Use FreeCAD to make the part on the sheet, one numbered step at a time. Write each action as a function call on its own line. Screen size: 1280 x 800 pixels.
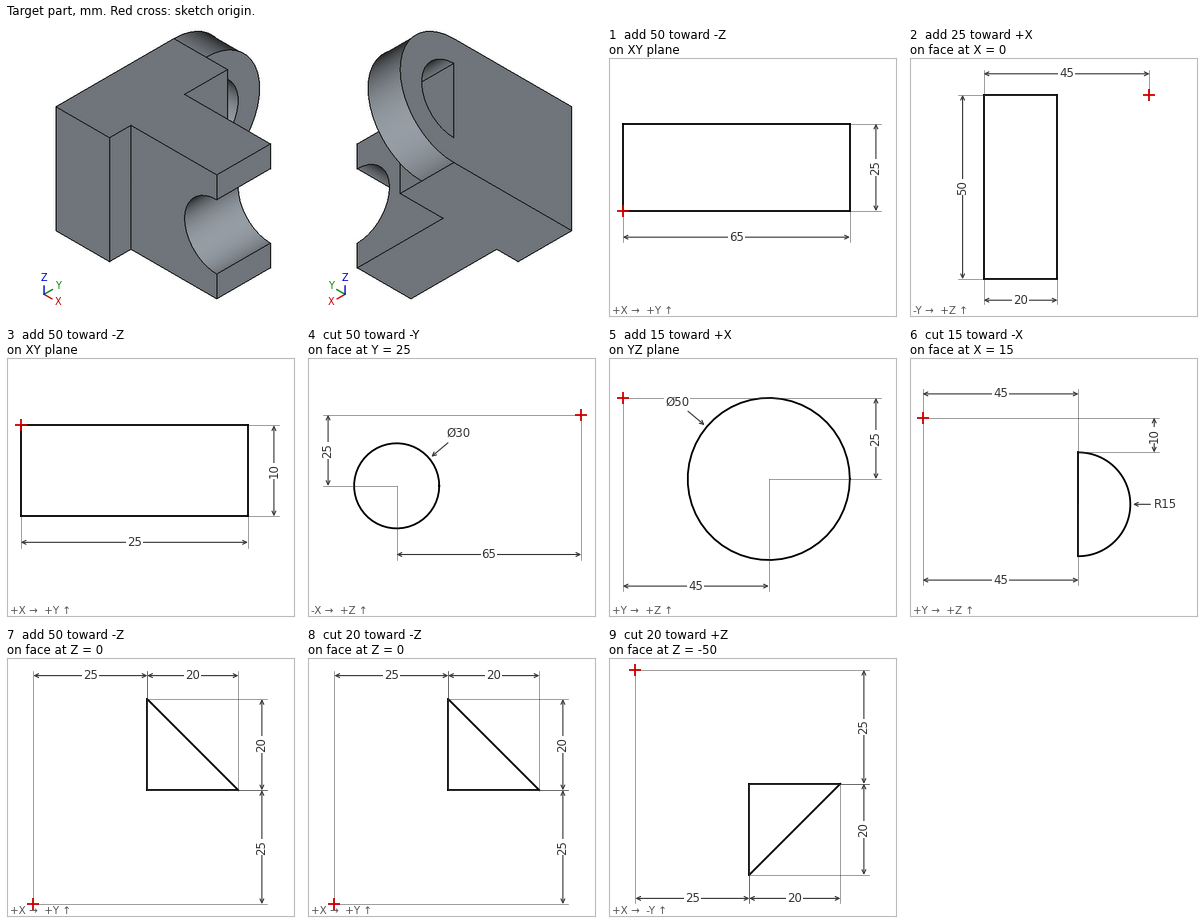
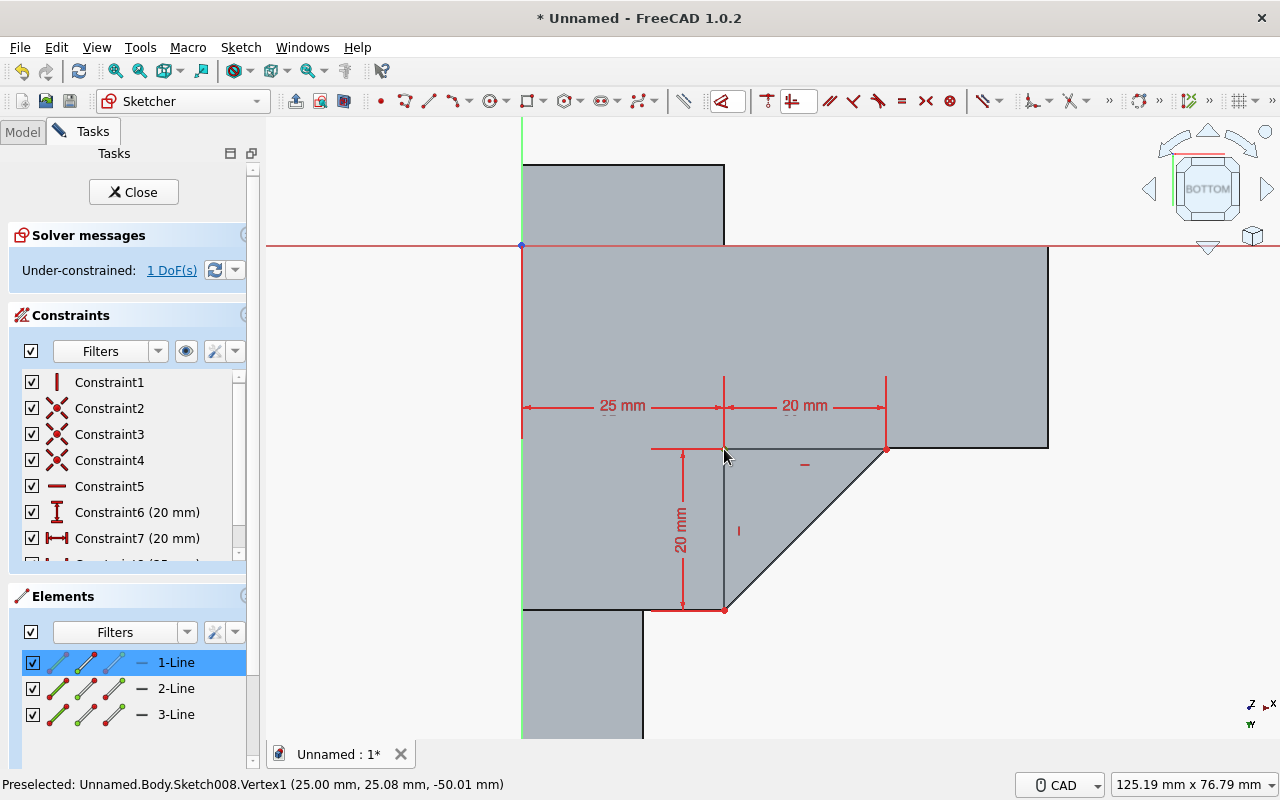
key(i)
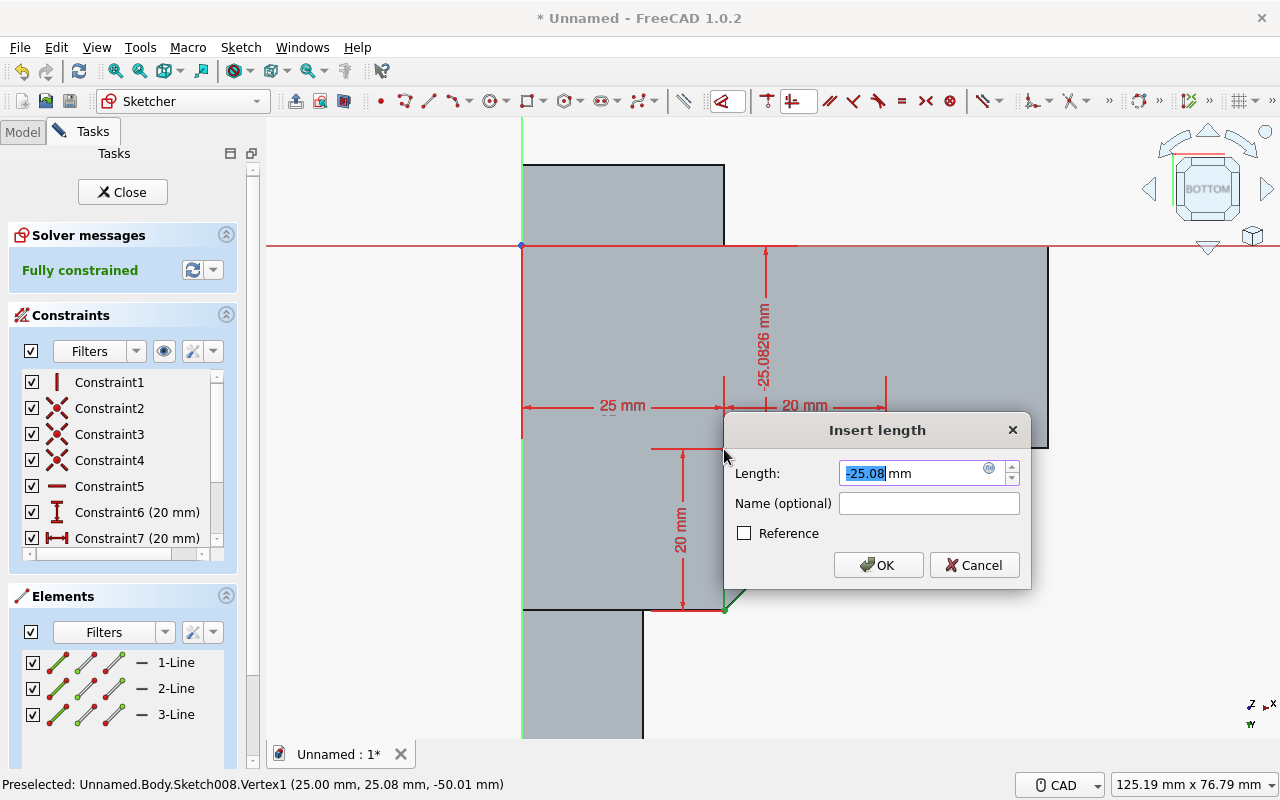
text(-25)
key(Return)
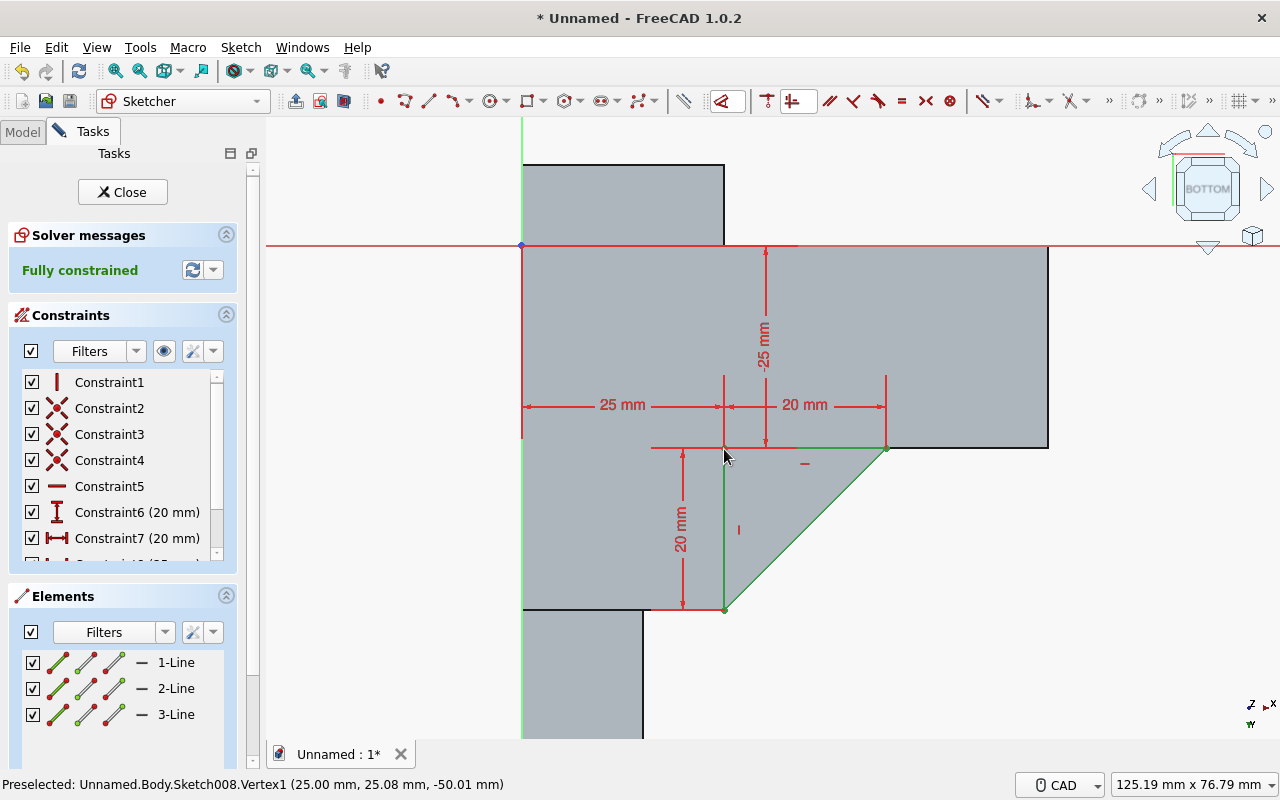
click(123, 192)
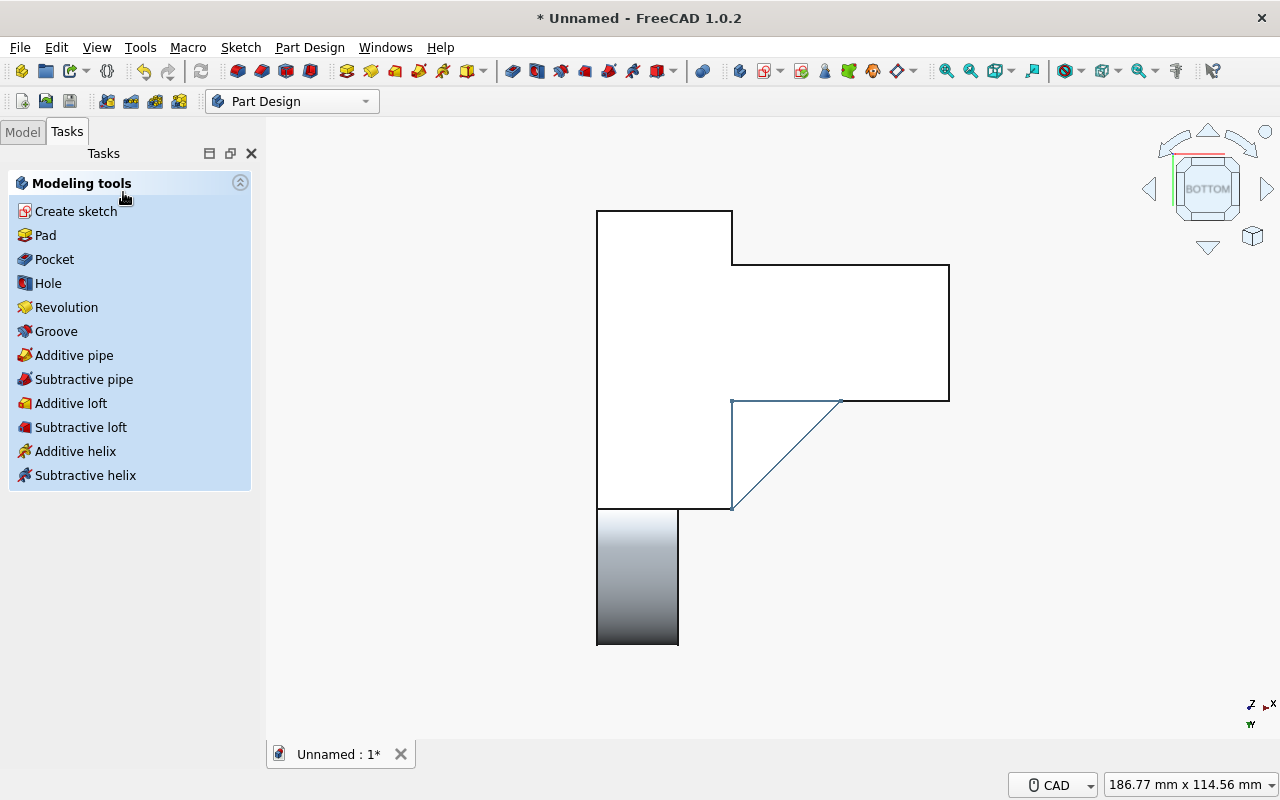
click(514, 72)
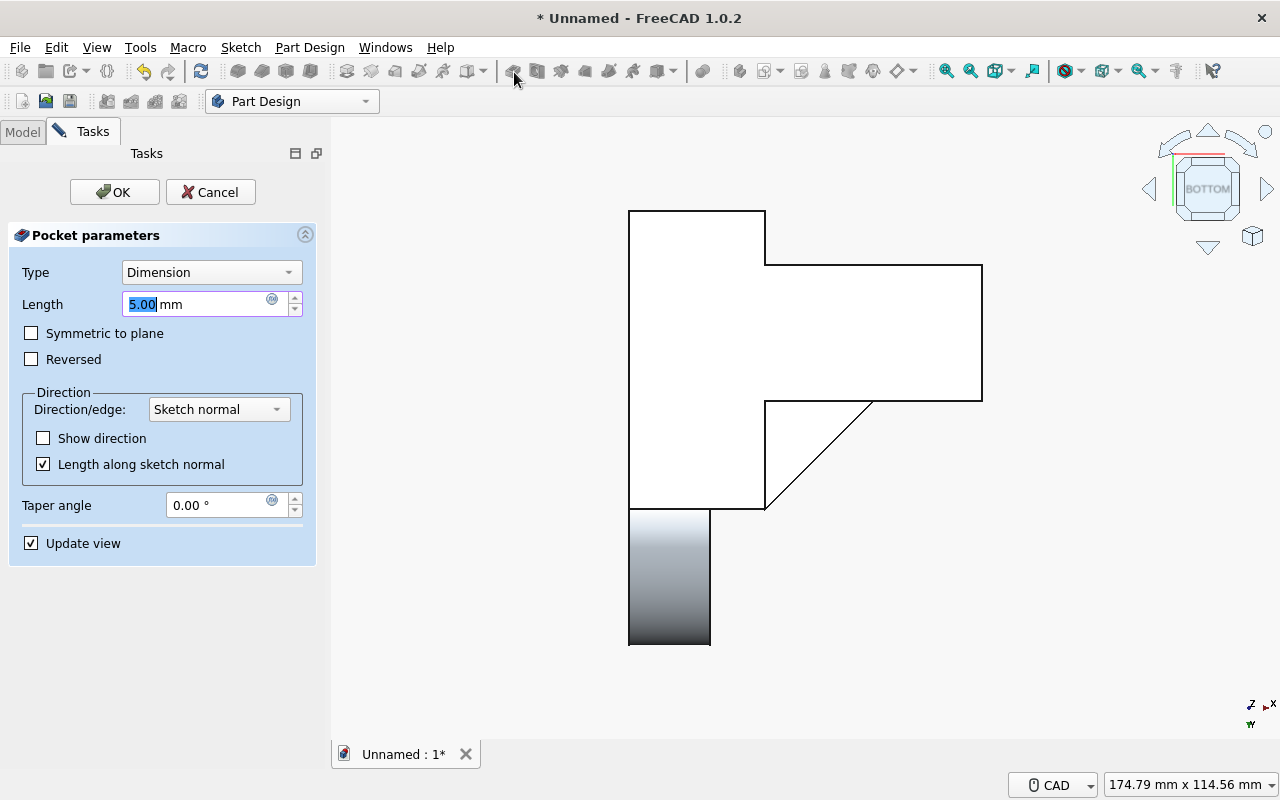
text(20)
key(Tab)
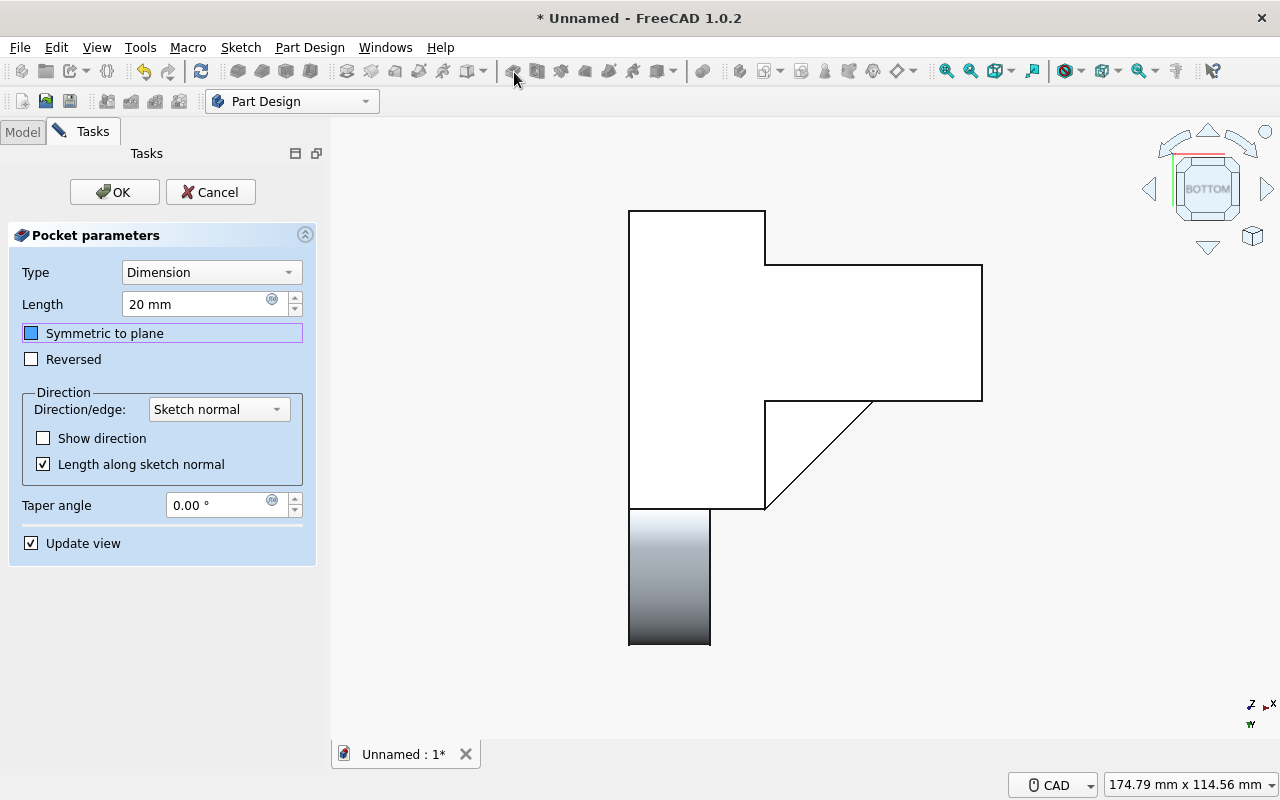
click(115, 192)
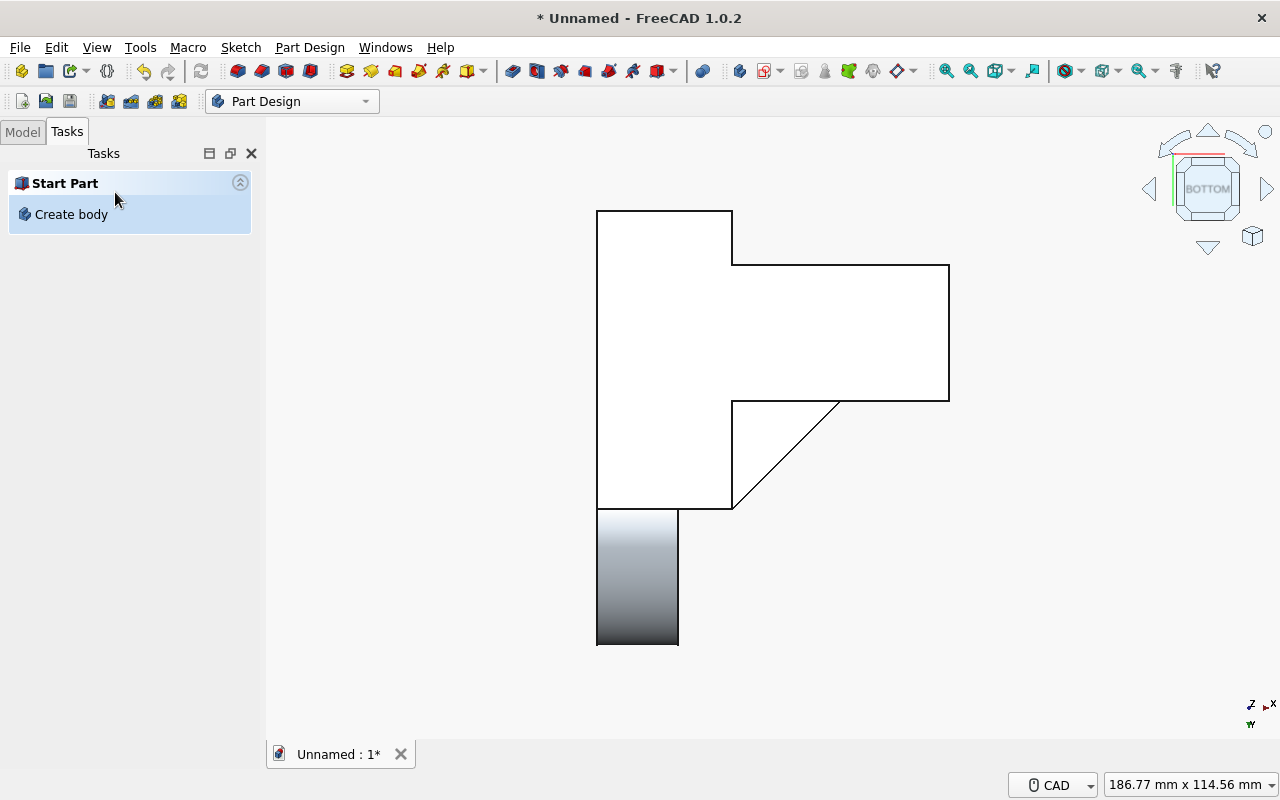
key(0)